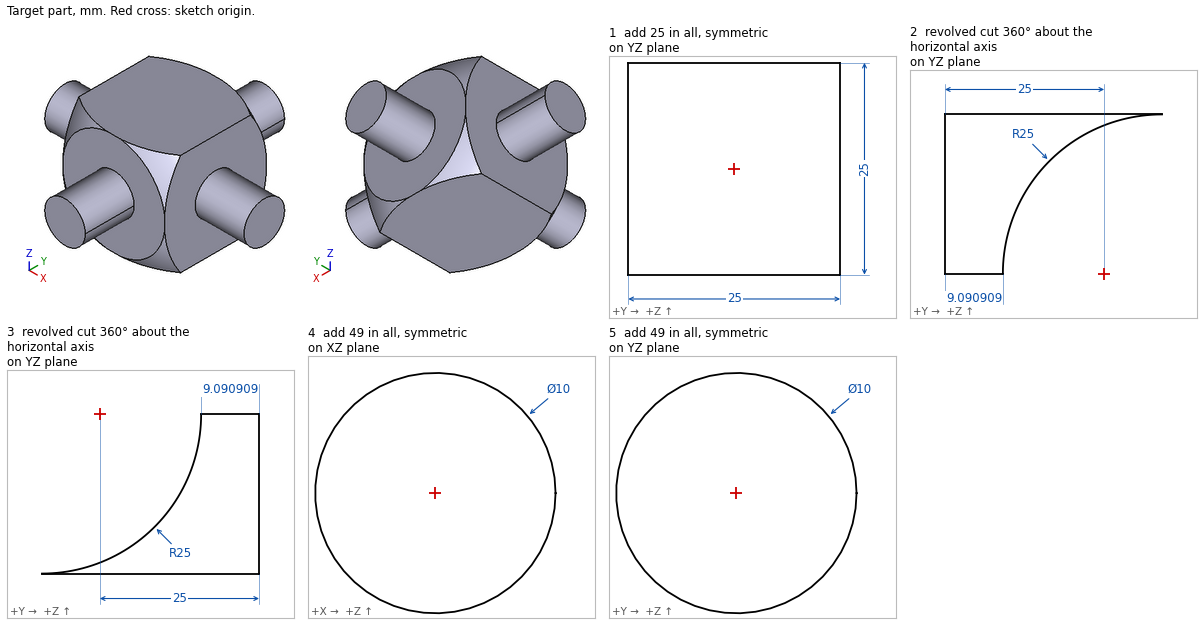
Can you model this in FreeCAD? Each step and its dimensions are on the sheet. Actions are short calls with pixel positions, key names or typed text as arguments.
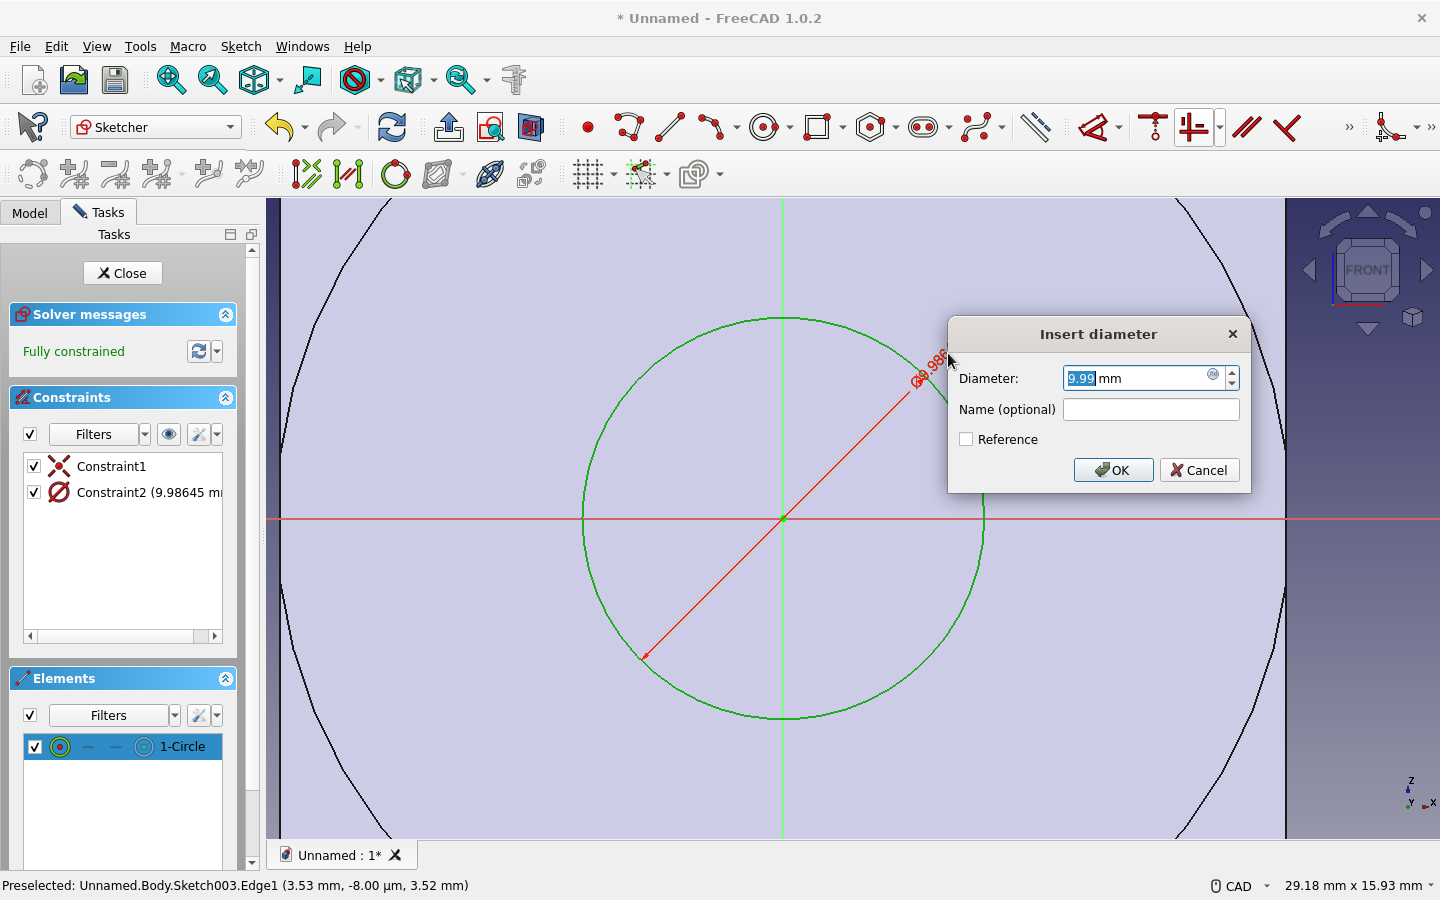
text(10)
key(Return)
key(Escape)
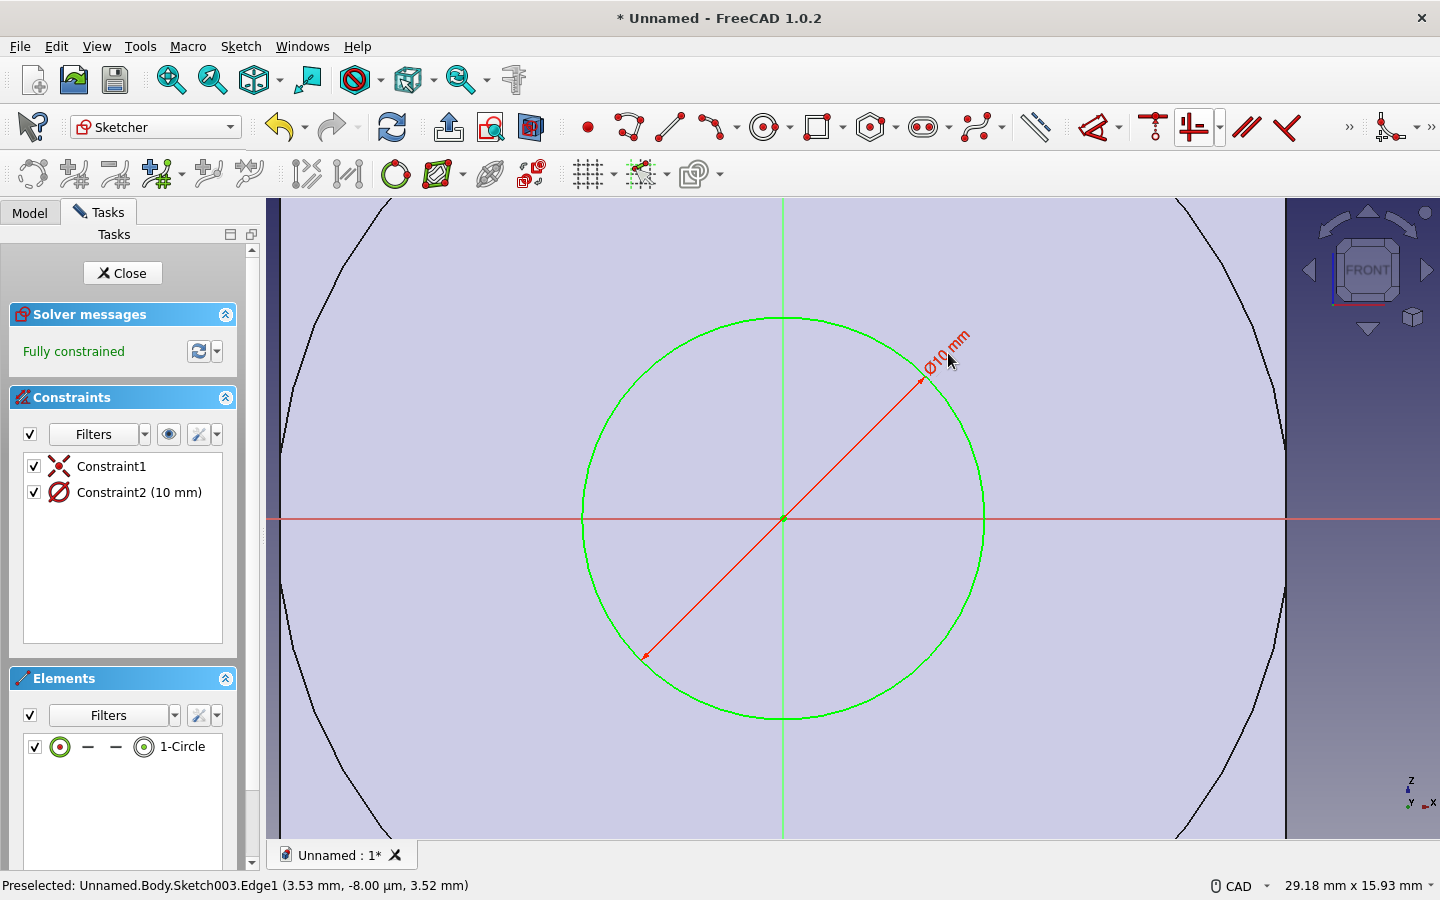
click(123, 273)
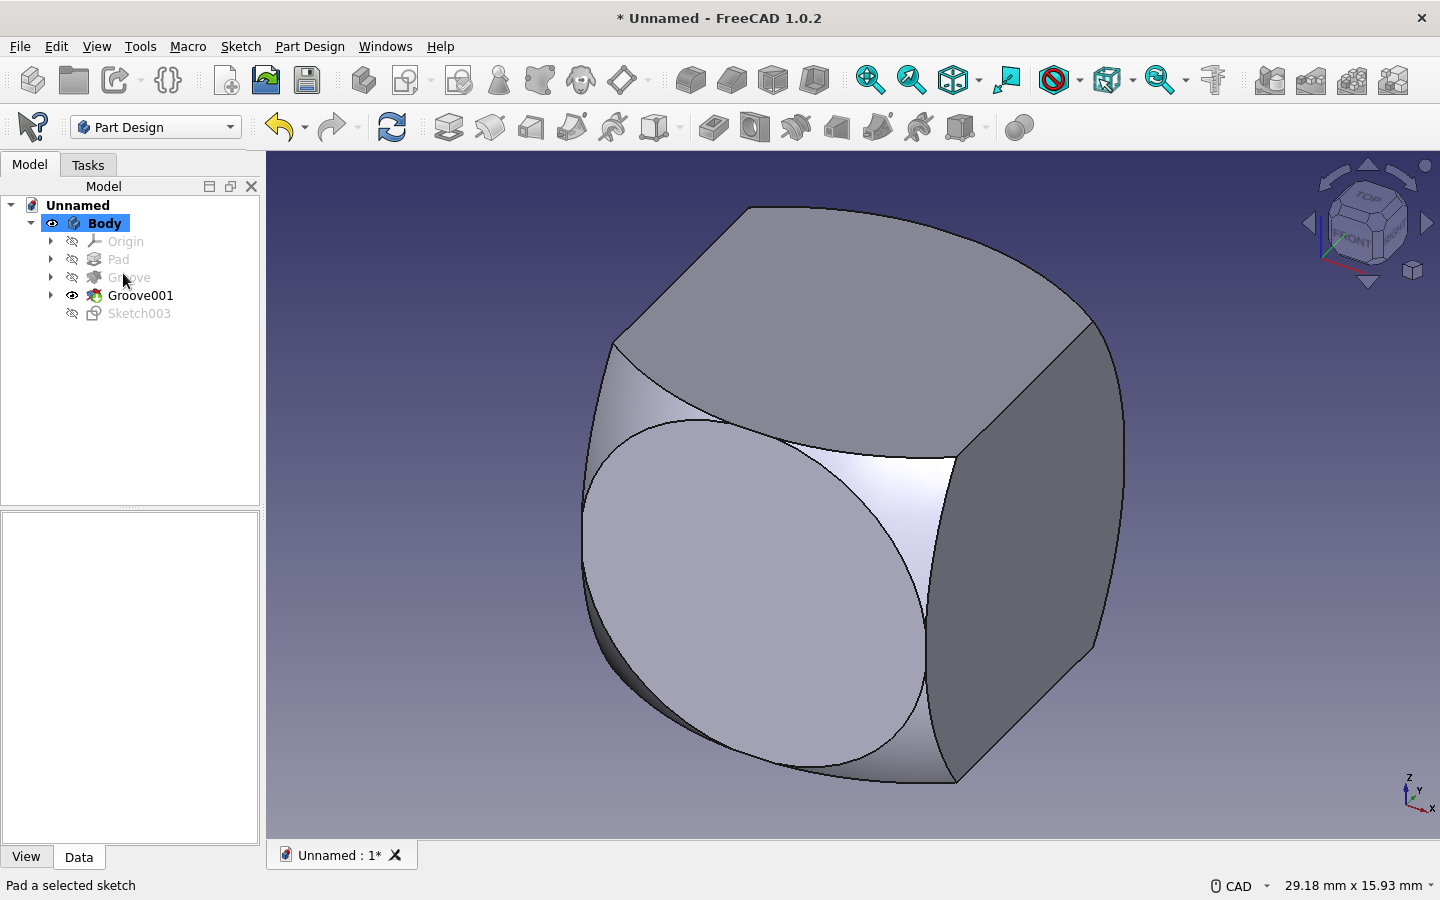
click(449, 128)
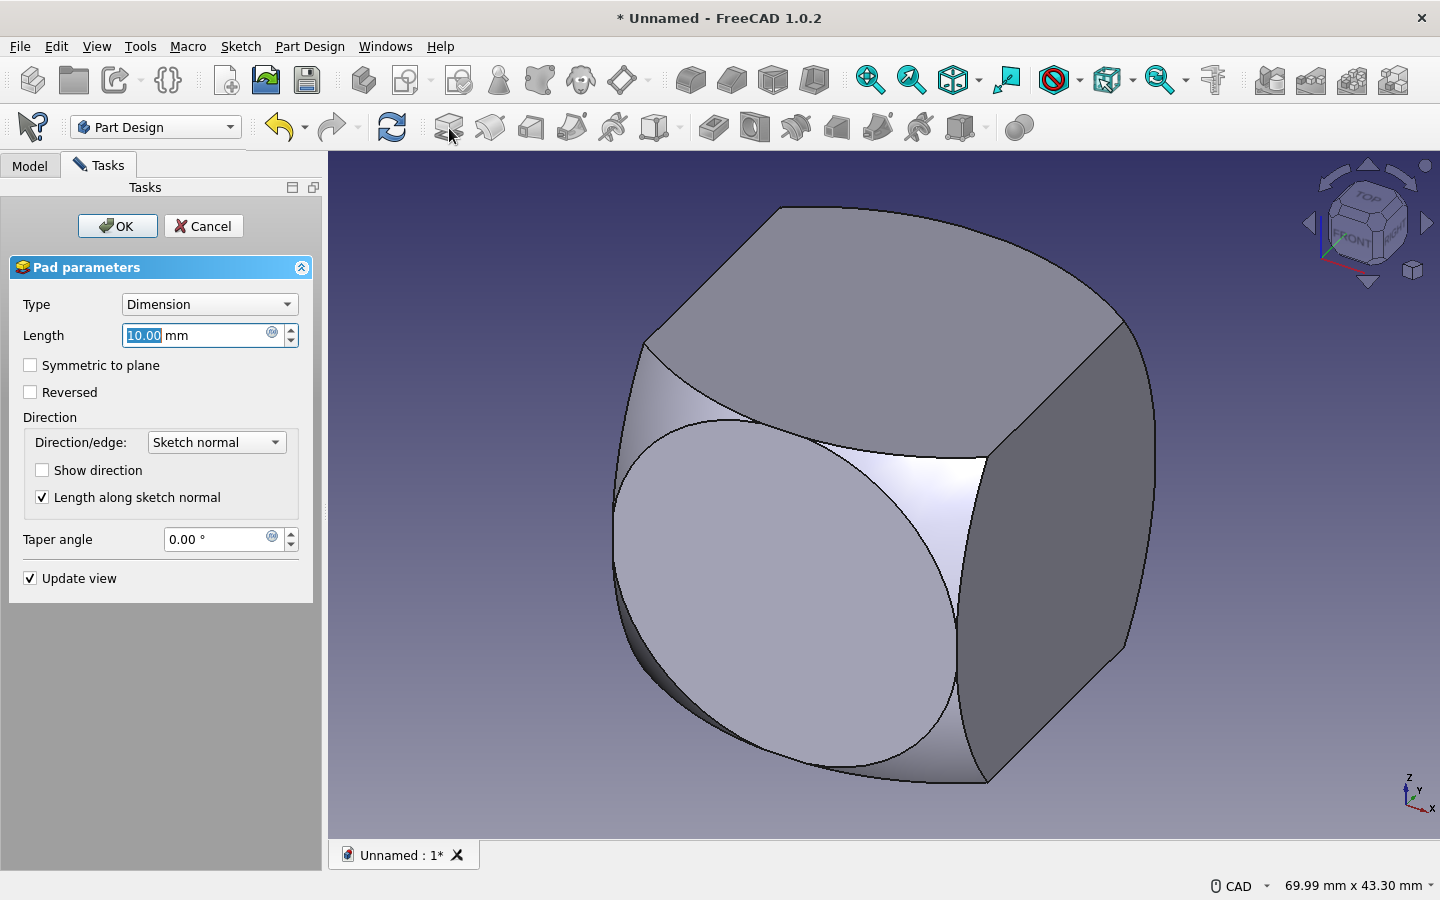
text(49)
key(Tab)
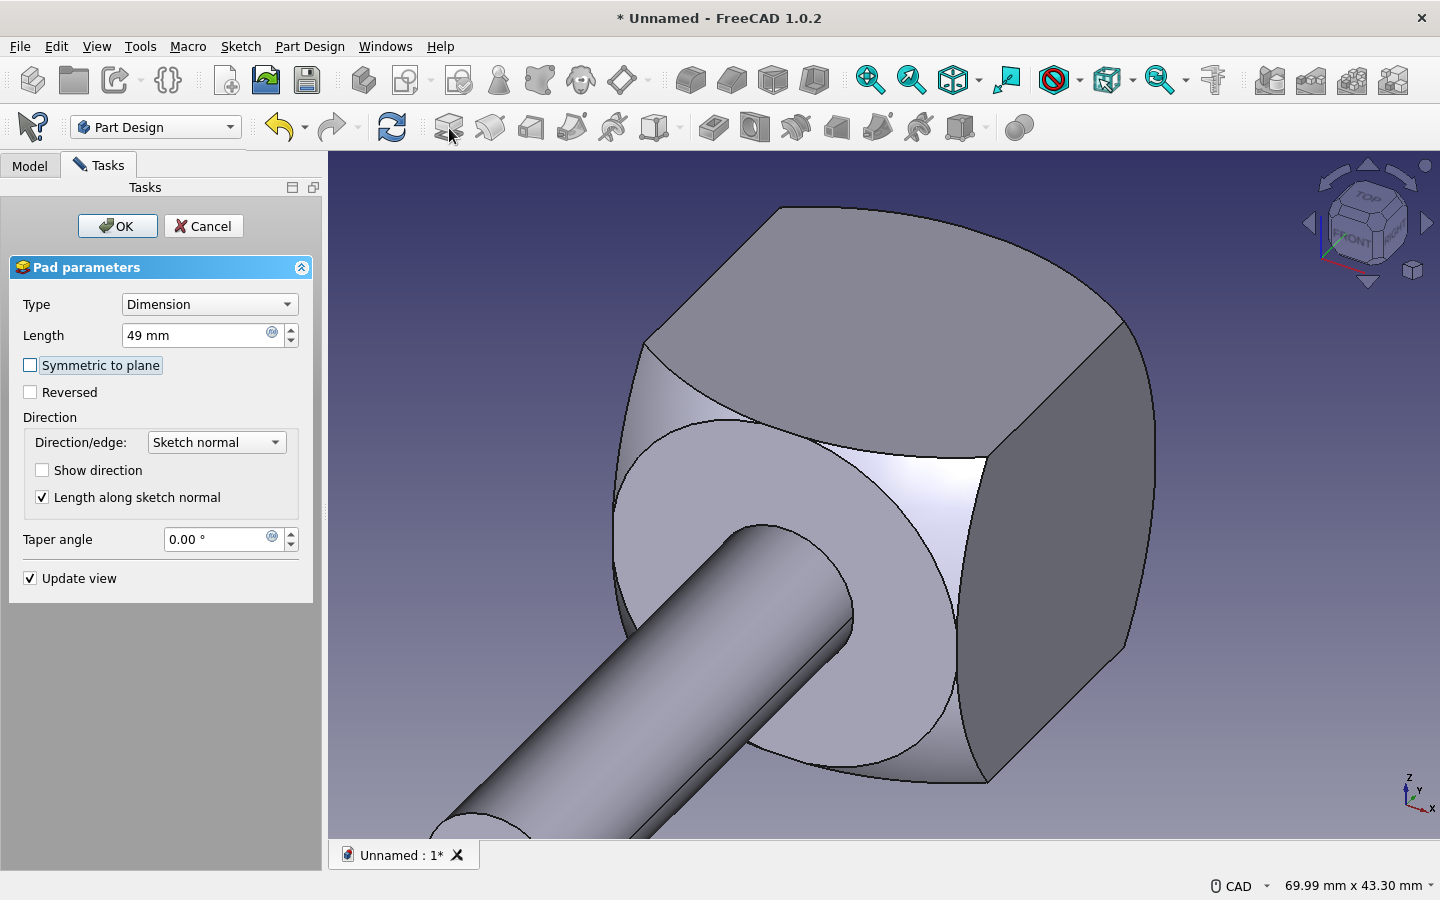
click(31, 365)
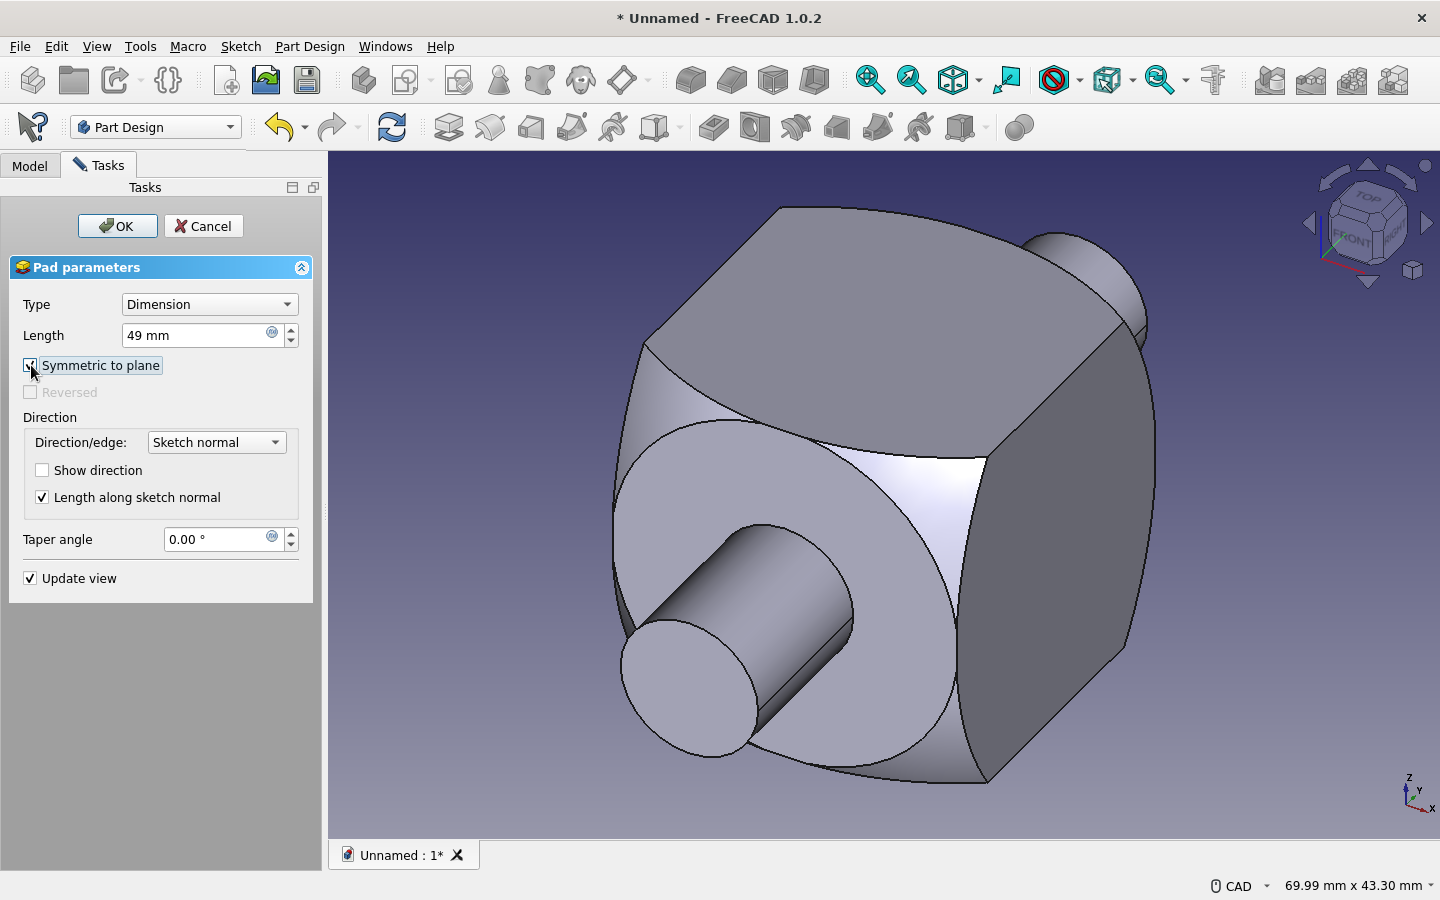
click(118, 226)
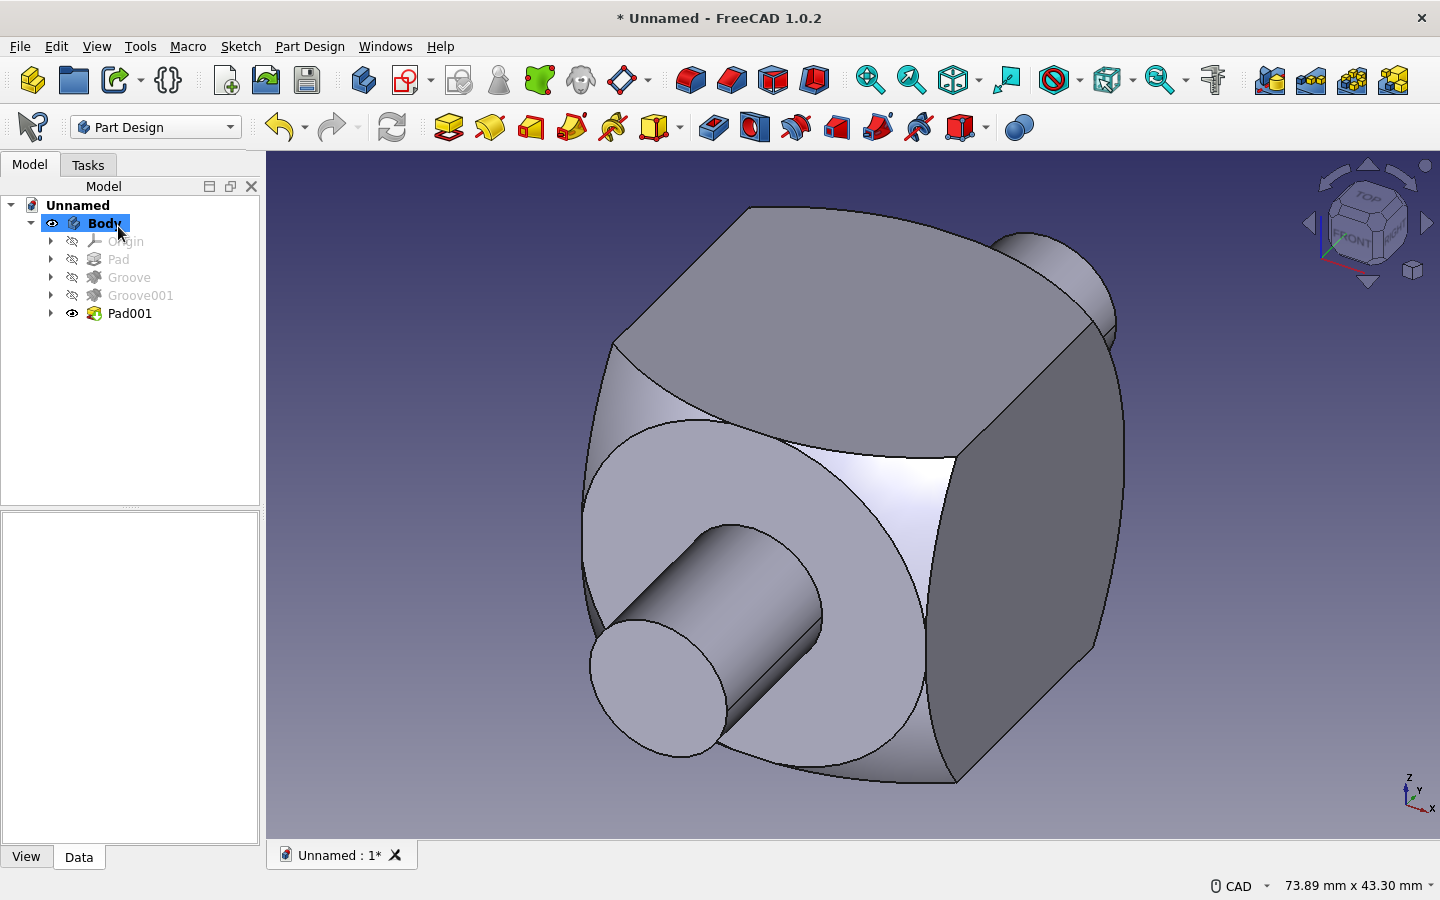
key(v)
key(f)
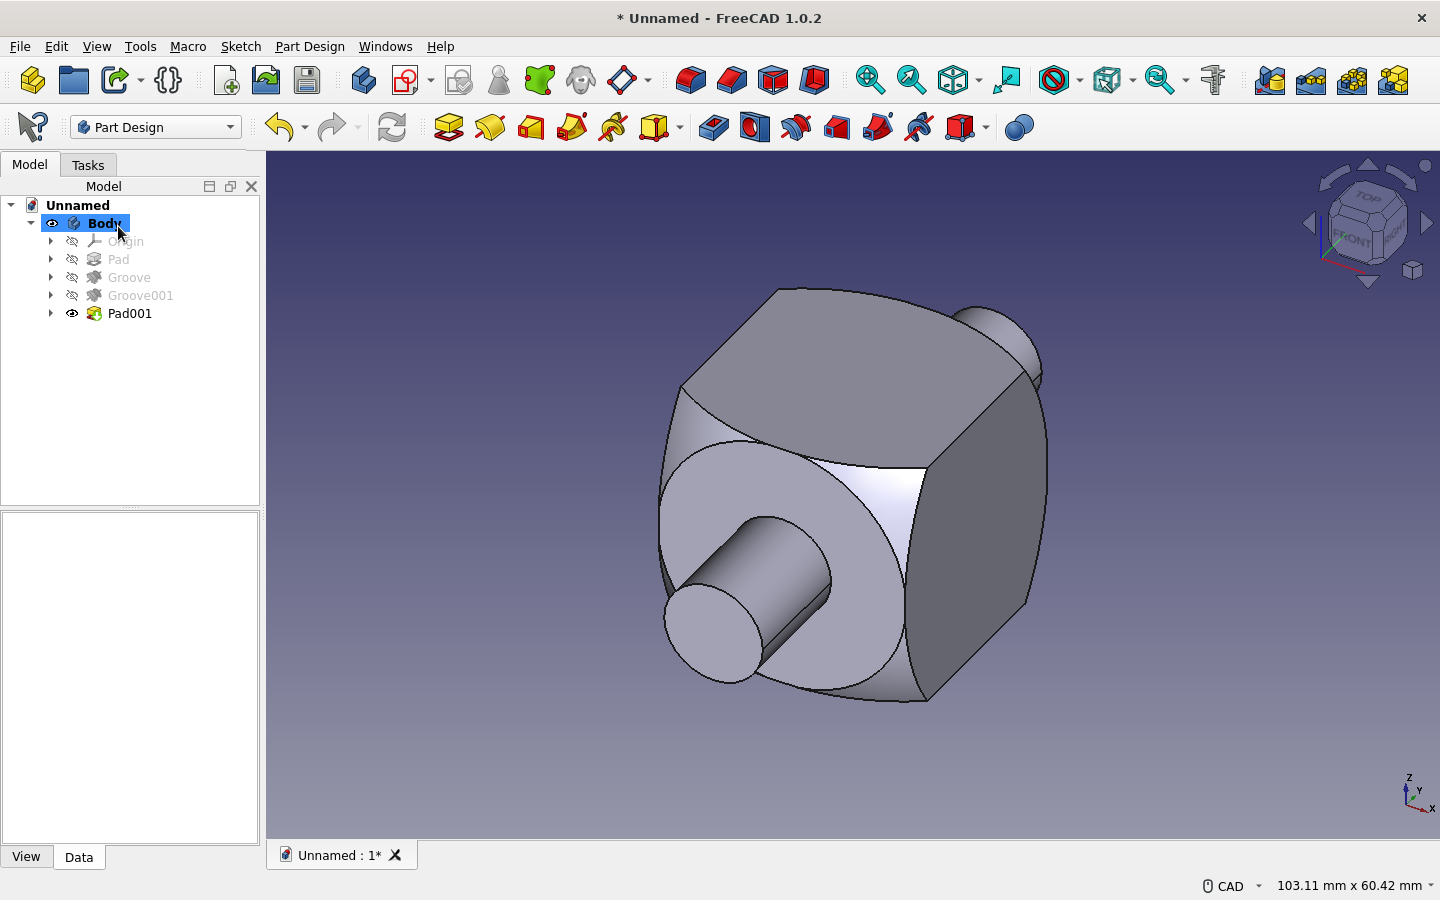
click(404, 80)